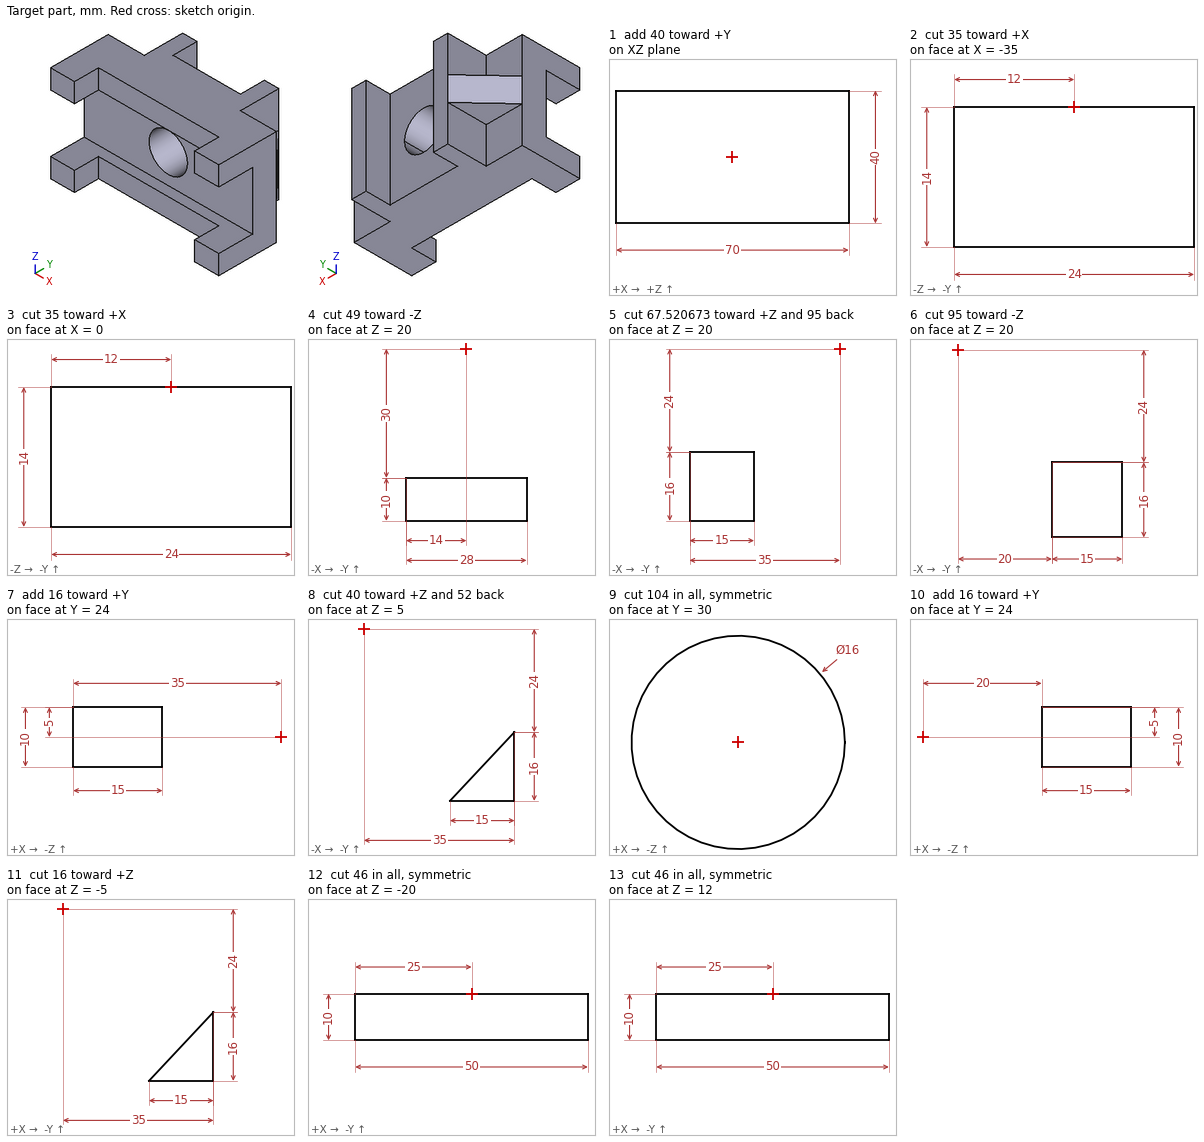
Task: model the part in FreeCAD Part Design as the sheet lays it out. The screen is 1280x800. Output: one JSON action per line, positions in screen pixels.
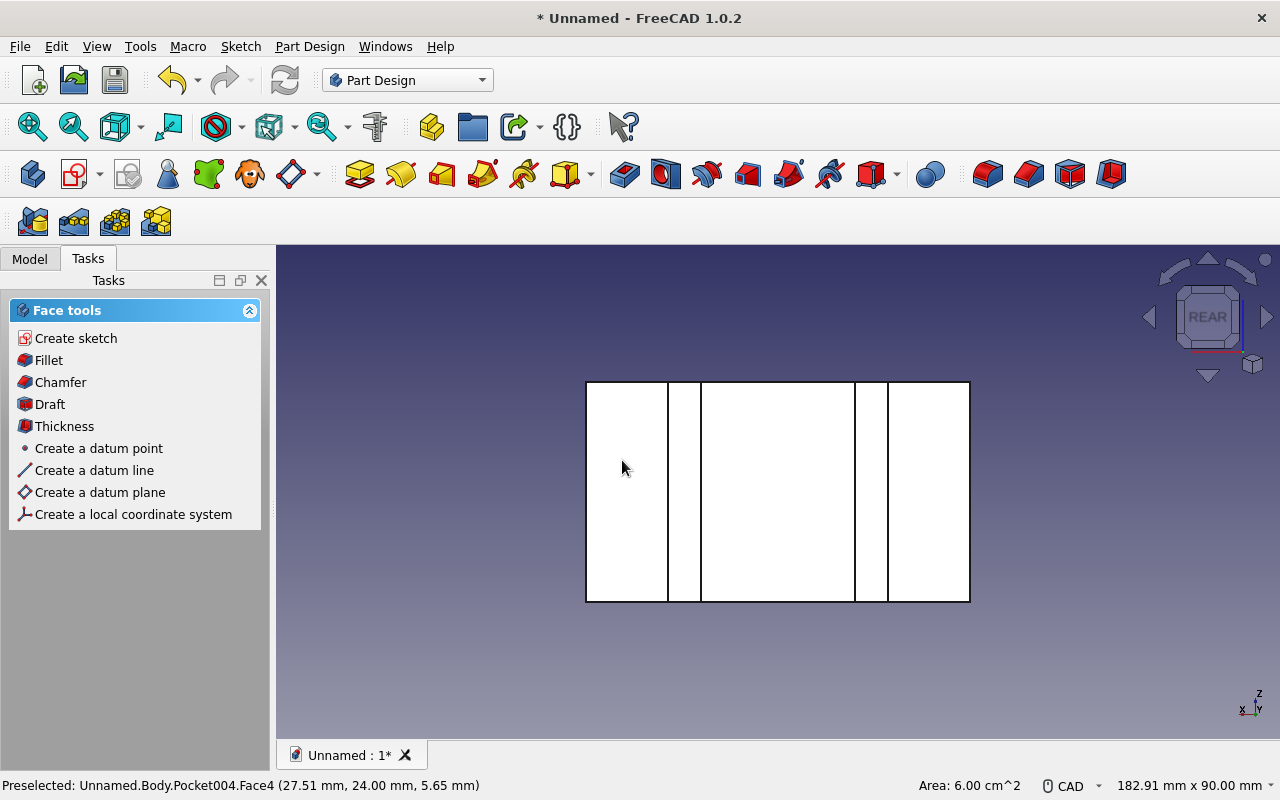
{"action": "left_click", "coordinate": [74, 174]}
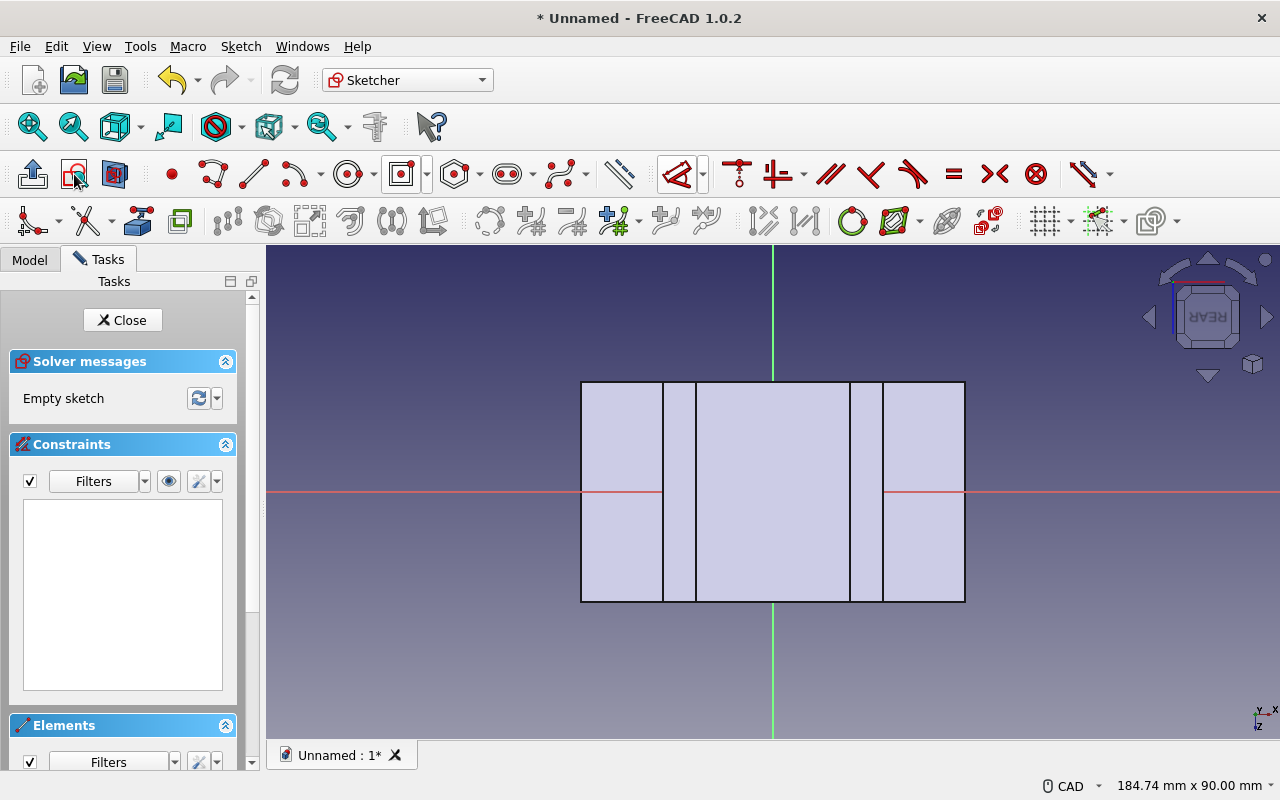
{"action": "key", "text": "q s"}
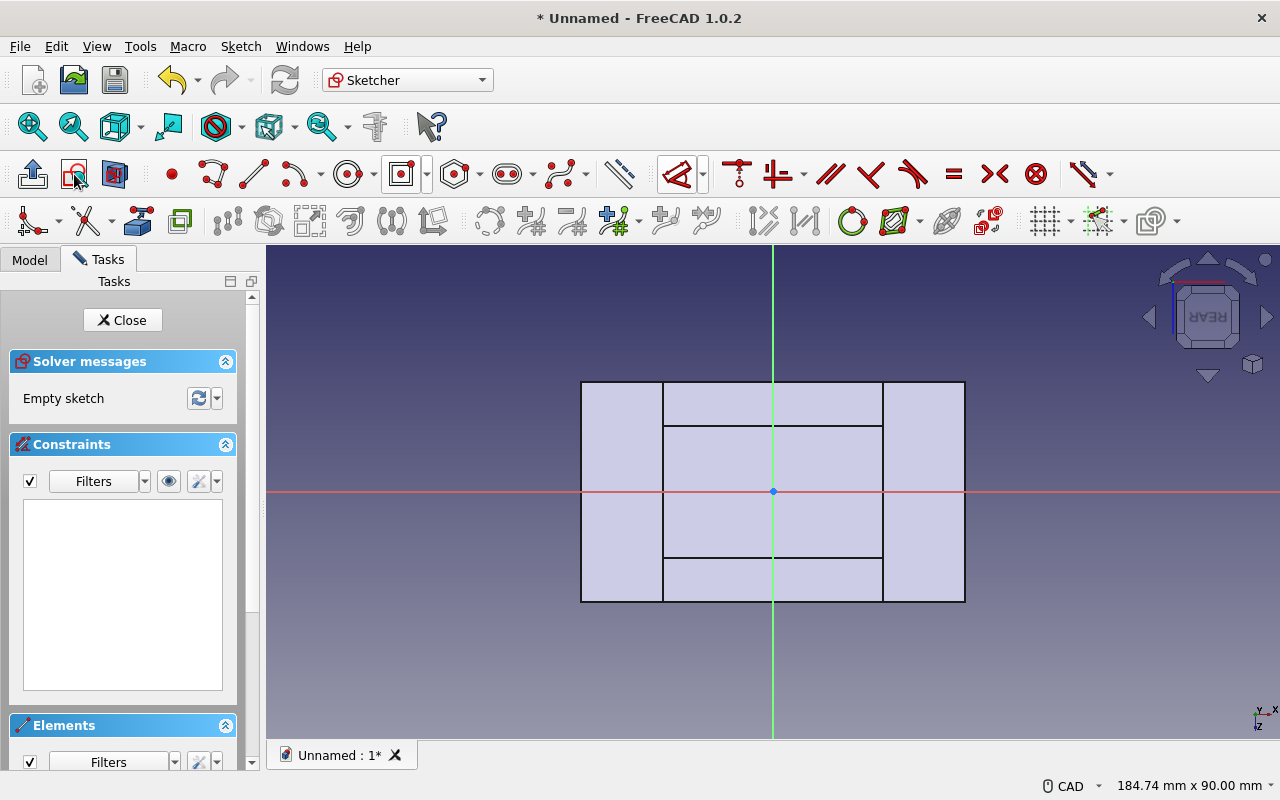
{"action": "scroll", "coordinate": [665, 492], "scroll_direction": "up", "scroll_amount": 6}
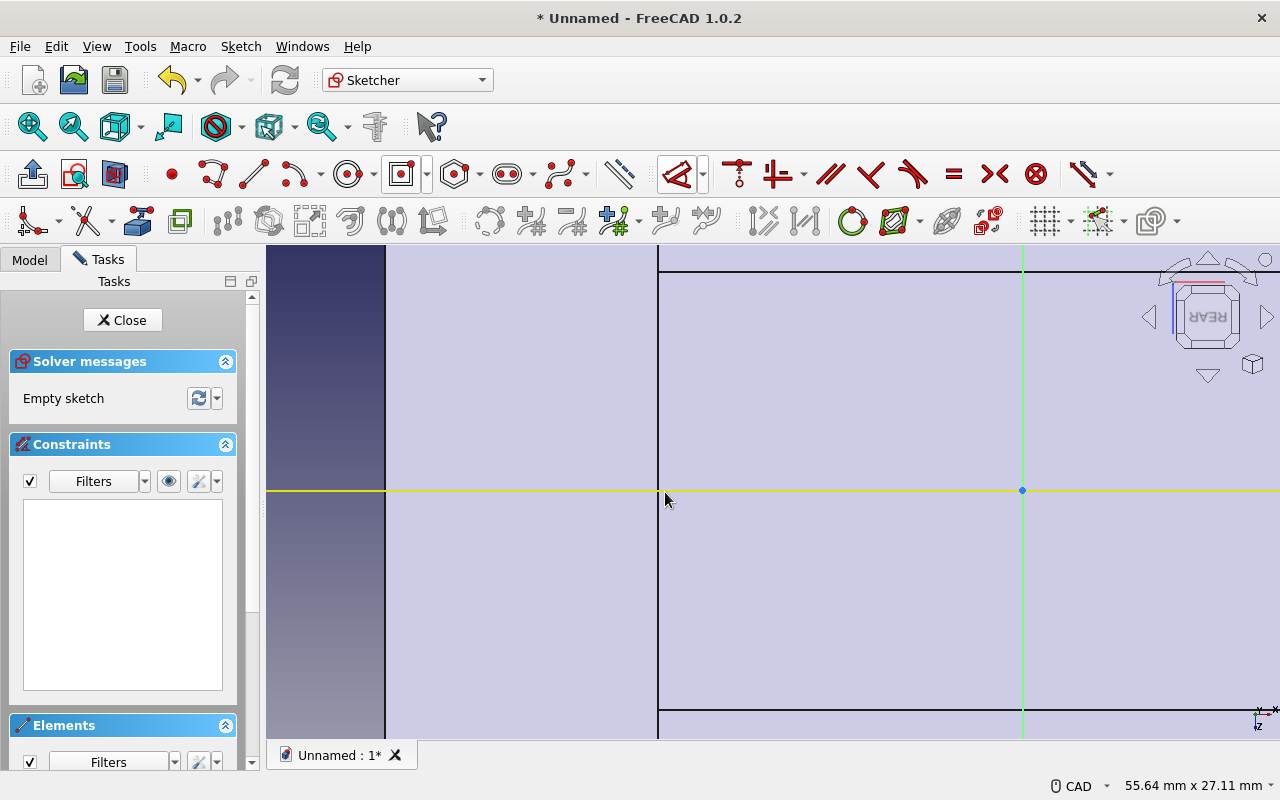
{"action": "left_click", "coordinate": [426, 174]}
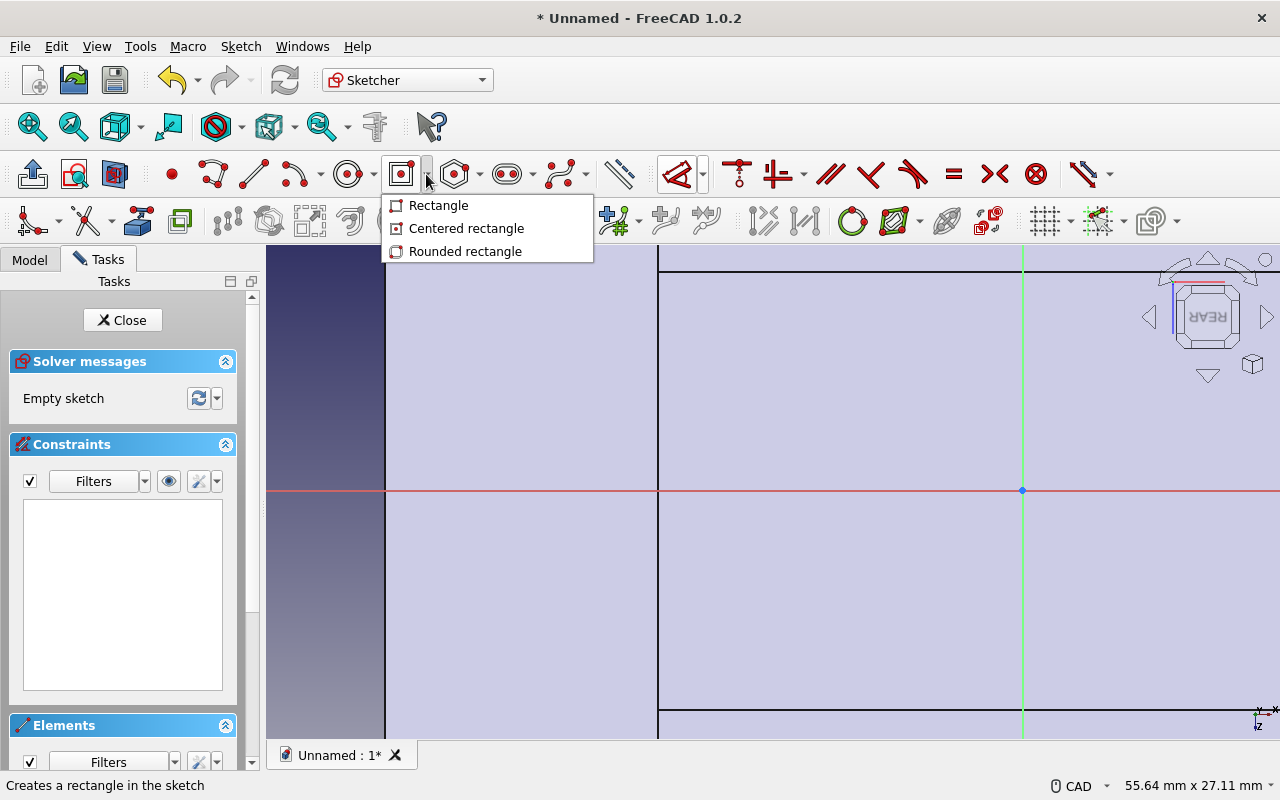
{"action": "left_click", "coordinate": [488, 206]}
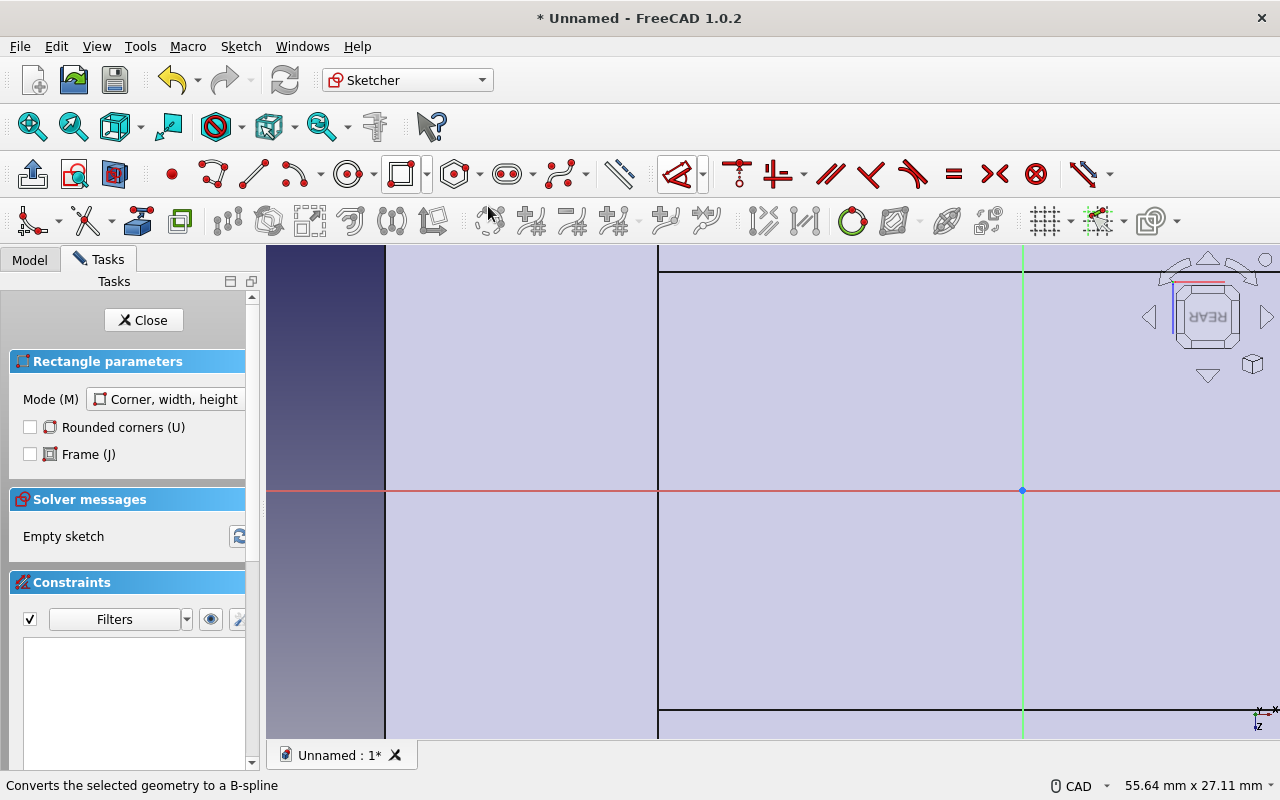
{"action": "left_click", "coordinate": [385, 400]}
{"action": "left_click", "coordinate": [658, 582]}
{"action": "key", "text": "Escape"}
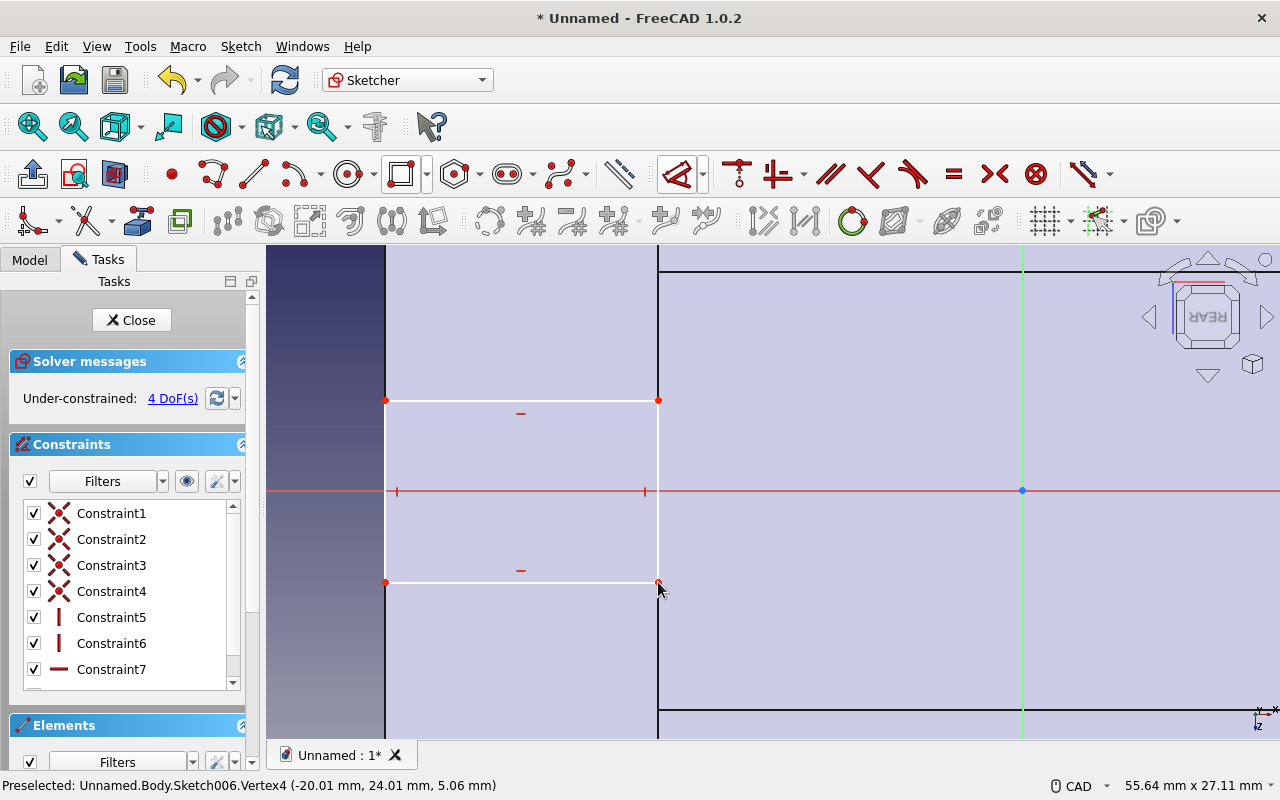
{"action": "left_click", "coordinate": [385, 456]}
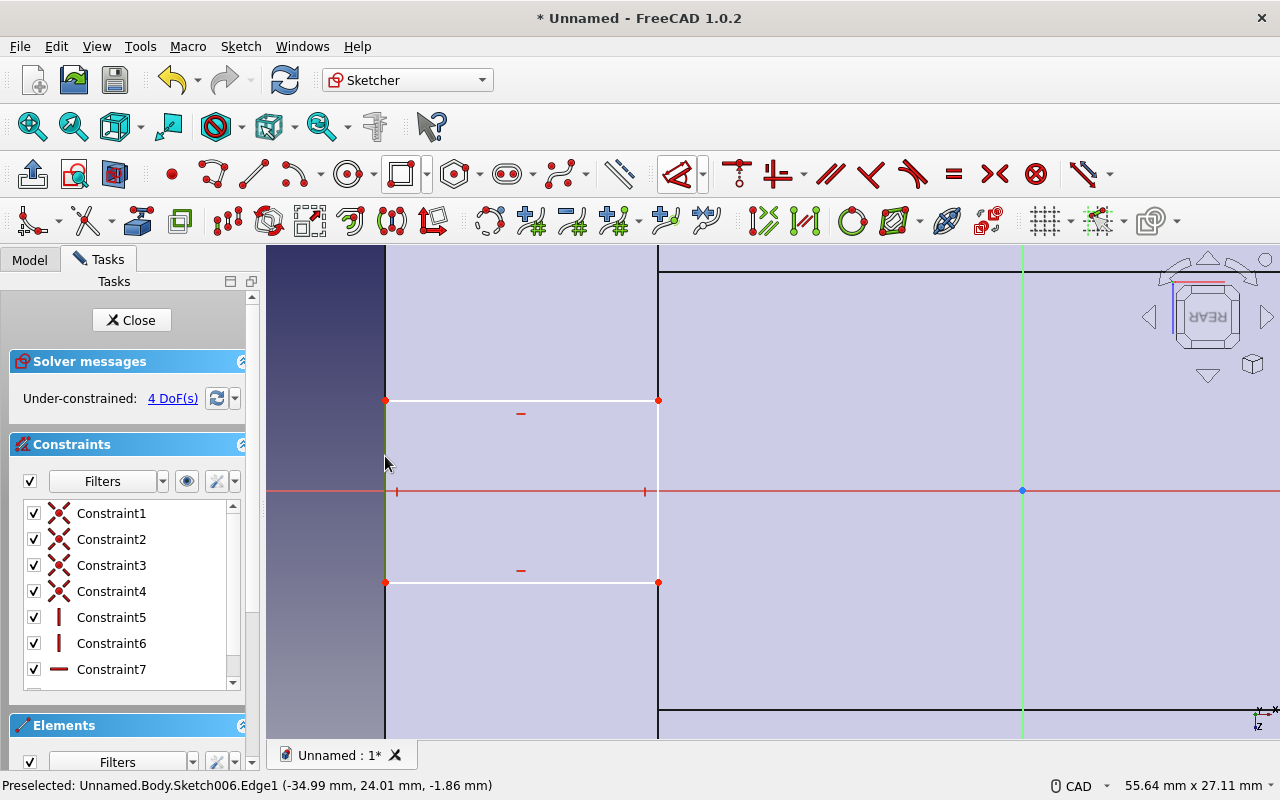
{"action": "left_click", "coordinate": [702, 174]}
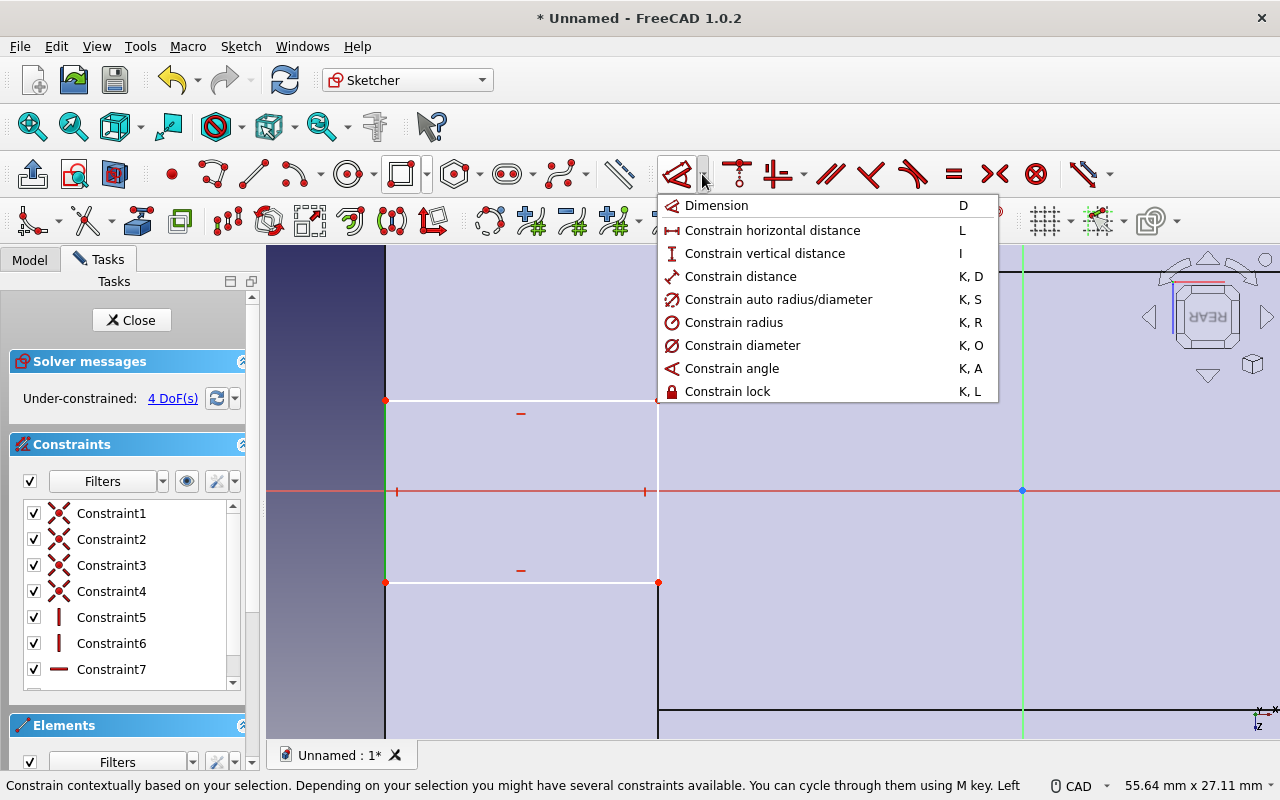
{"action": "left_click", "coordinate": [828, 254]}